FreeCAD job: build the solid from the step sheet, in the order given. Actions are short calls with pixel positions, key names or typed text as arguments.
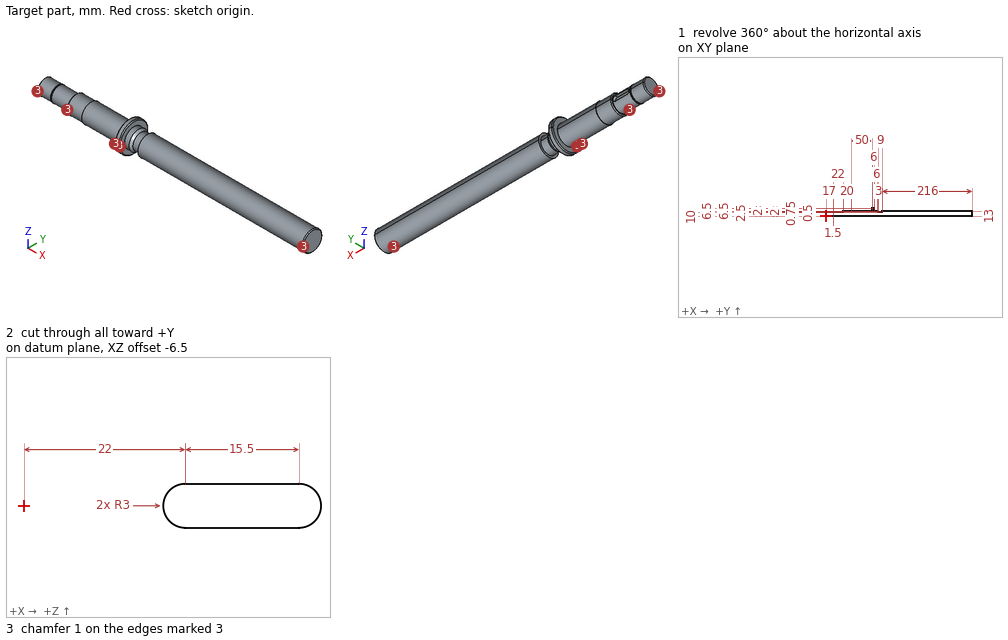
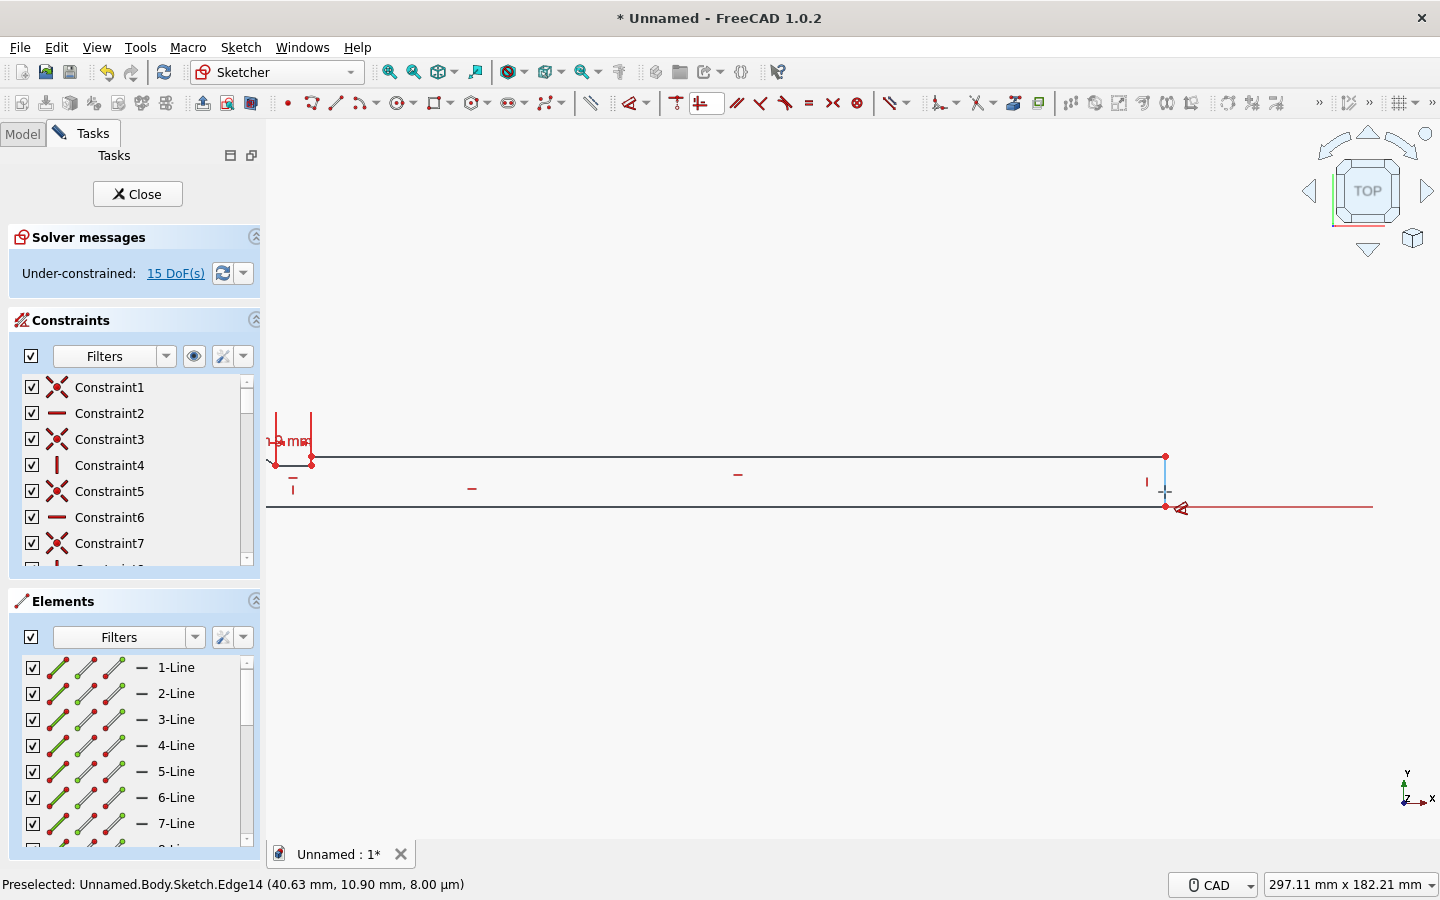
click(1165, 492)
click(1199, 482)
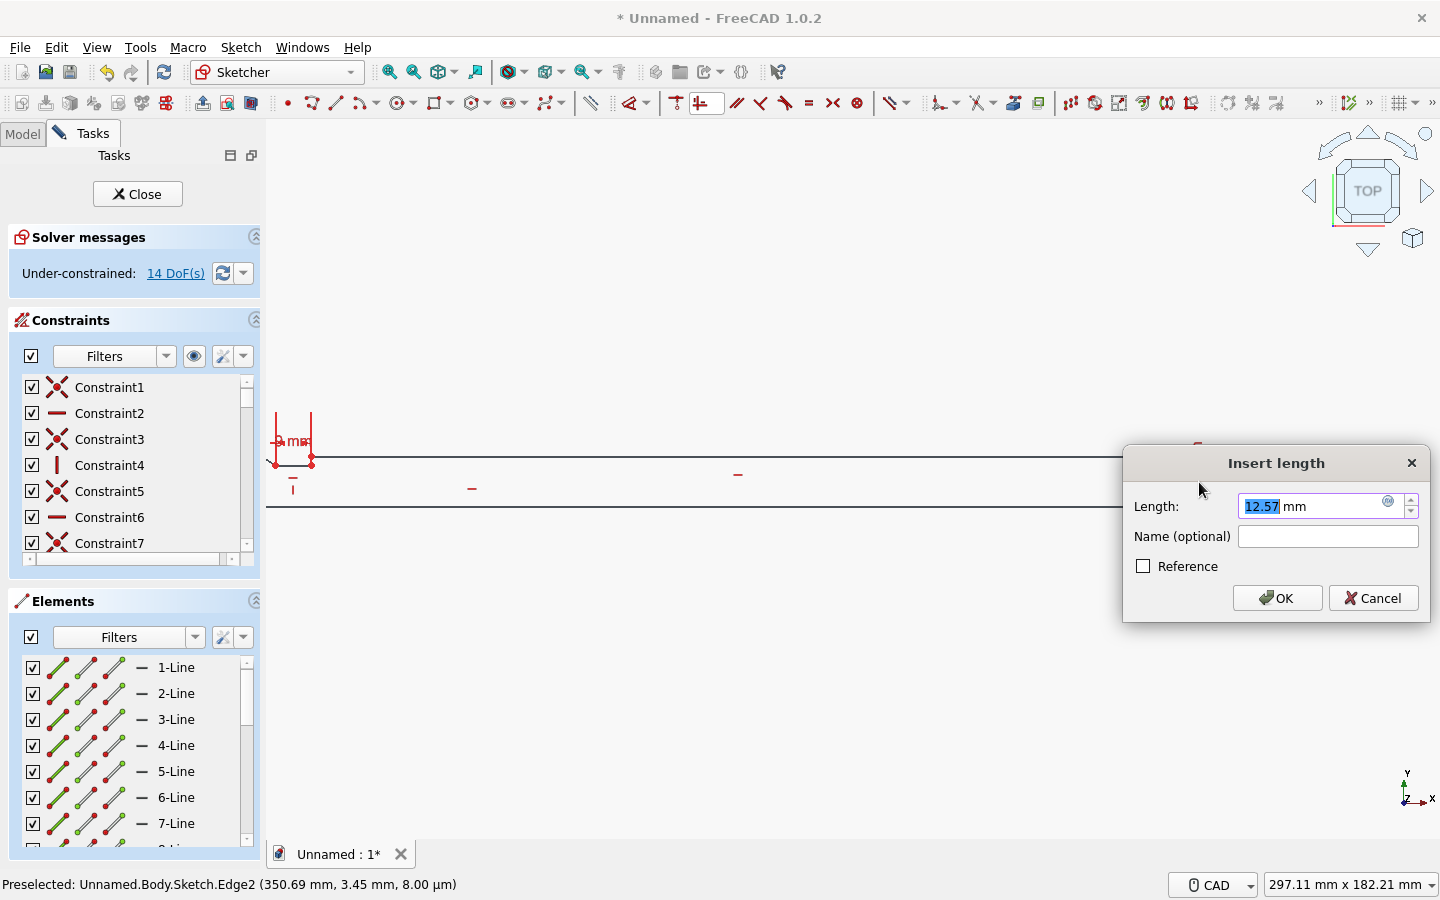
text(13)
key(Return)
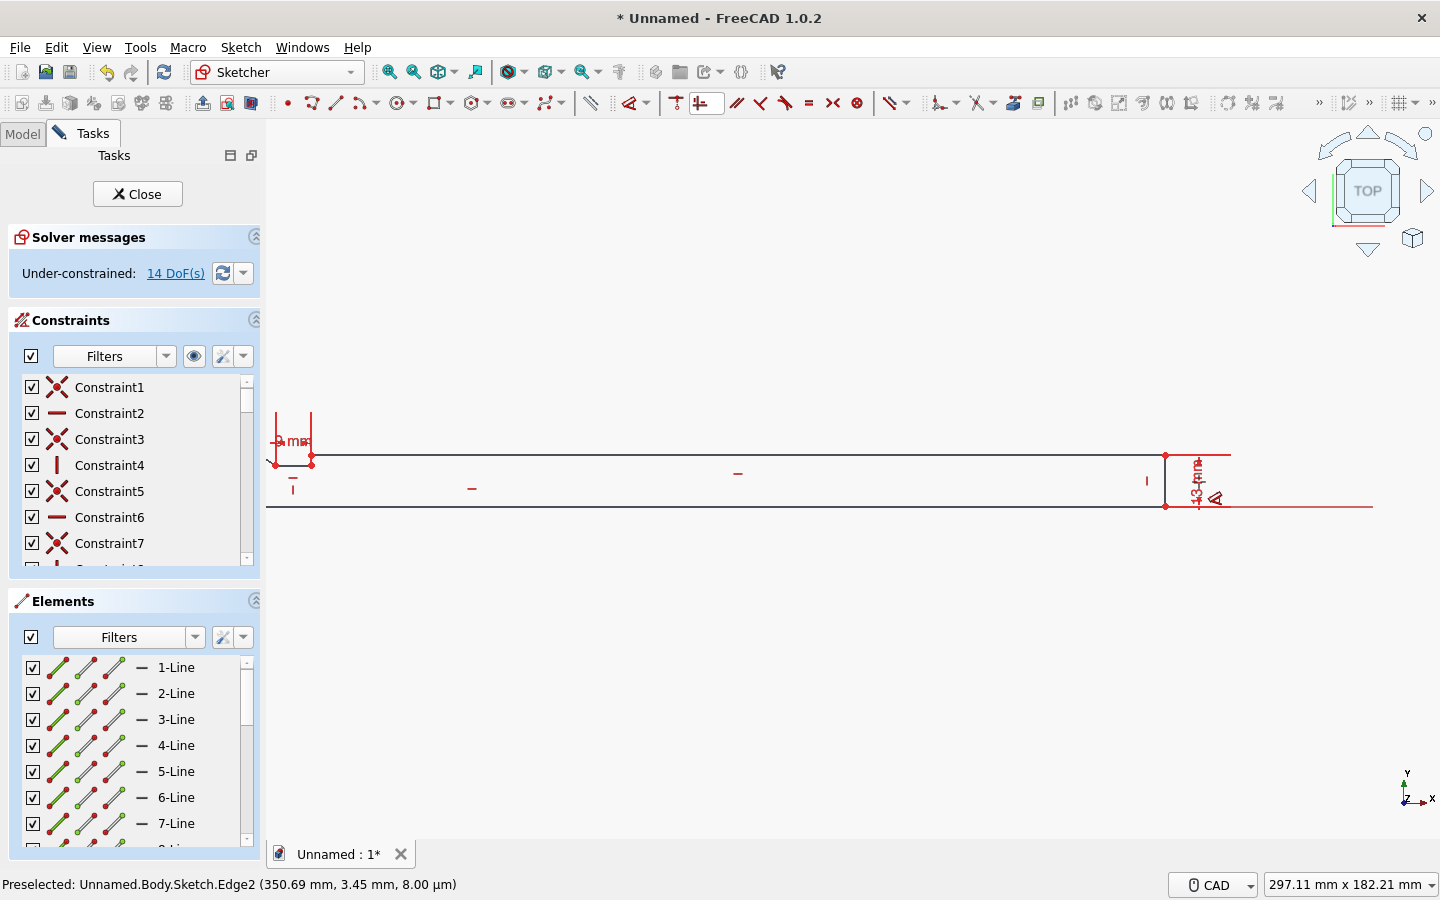
scroll(1165, 491, down, 3)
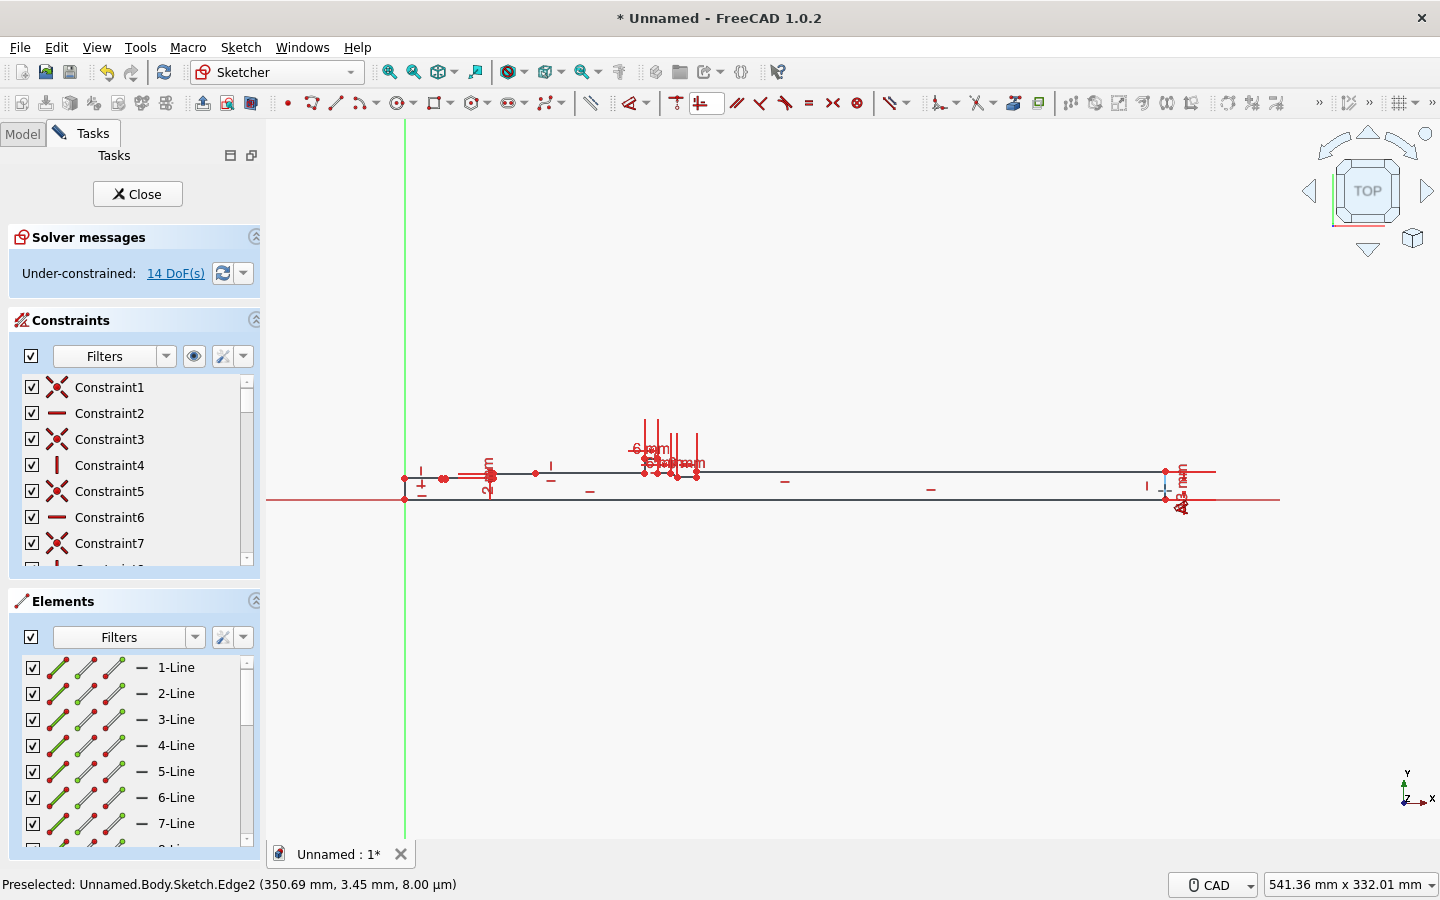
click(612, 473)
click(565, 439)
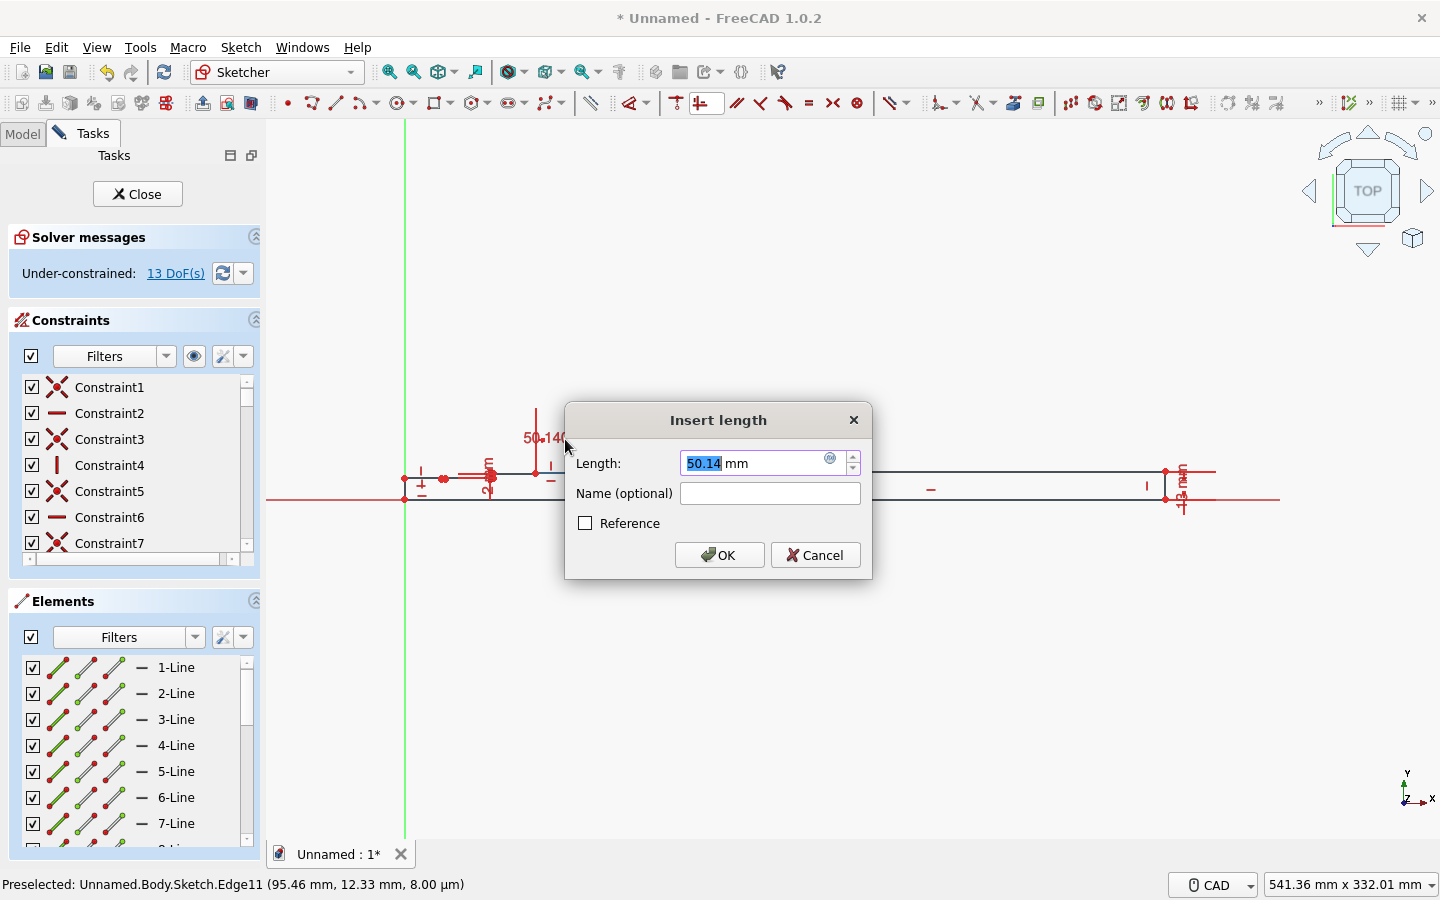
text(50)
key(Return)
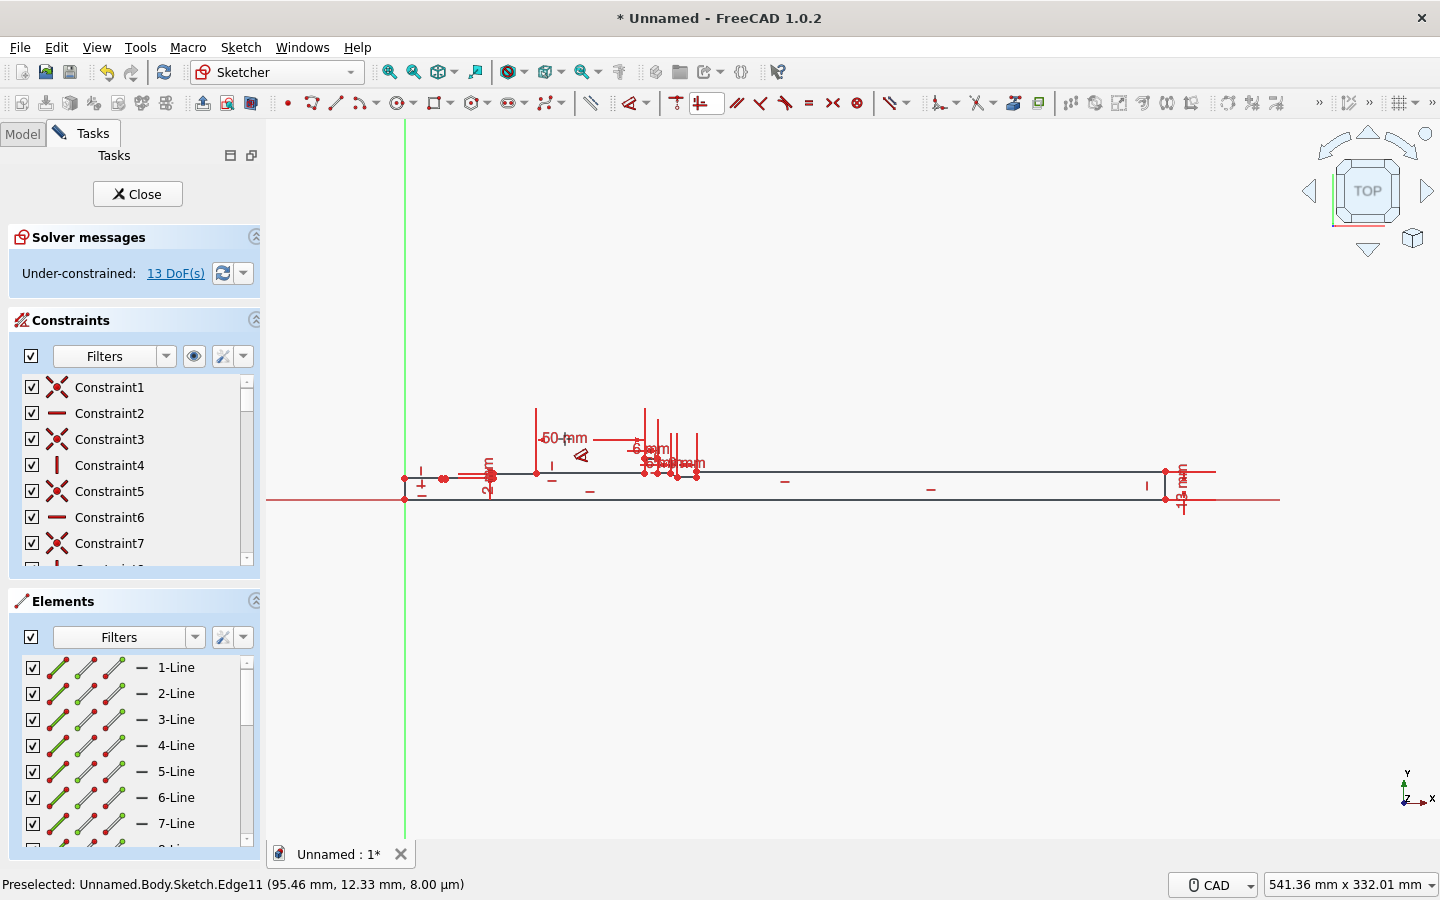
click(523, 474)
click(515, 416)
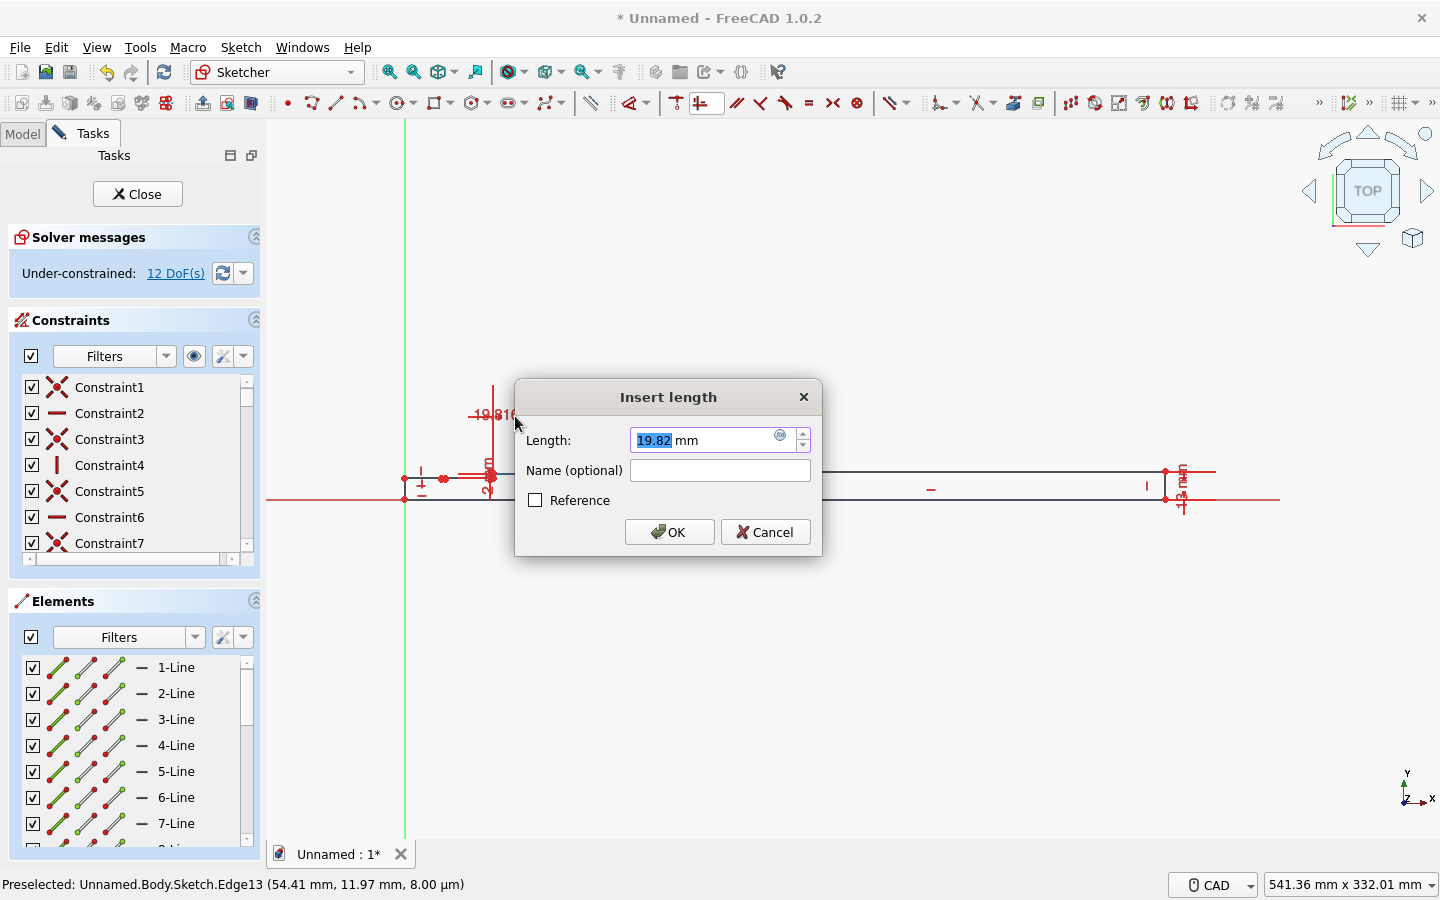
text(20)
key(Return)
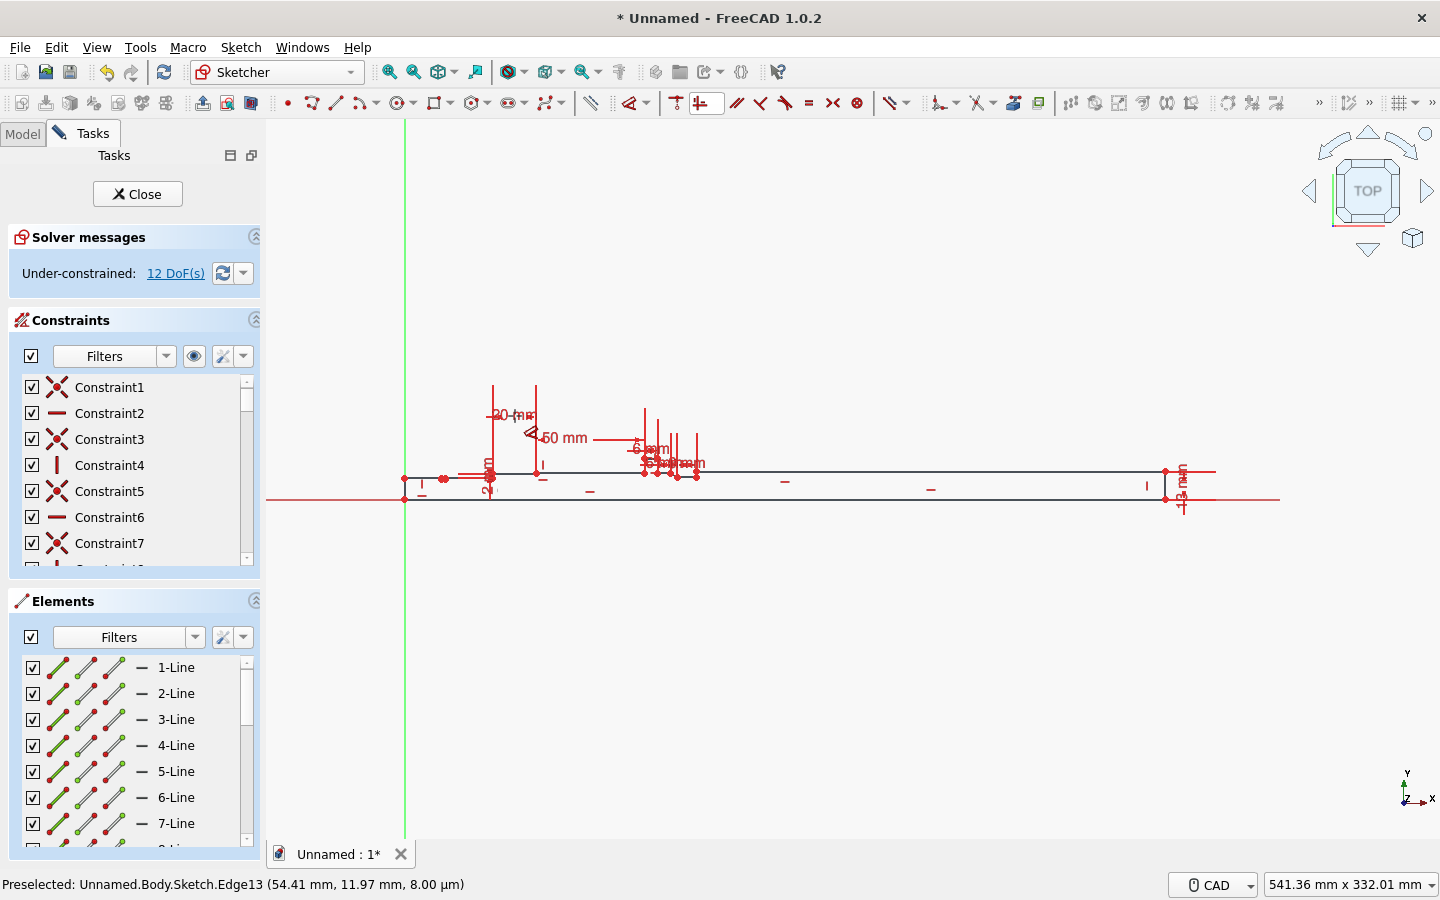
click(478, 478)
click(469, 444)